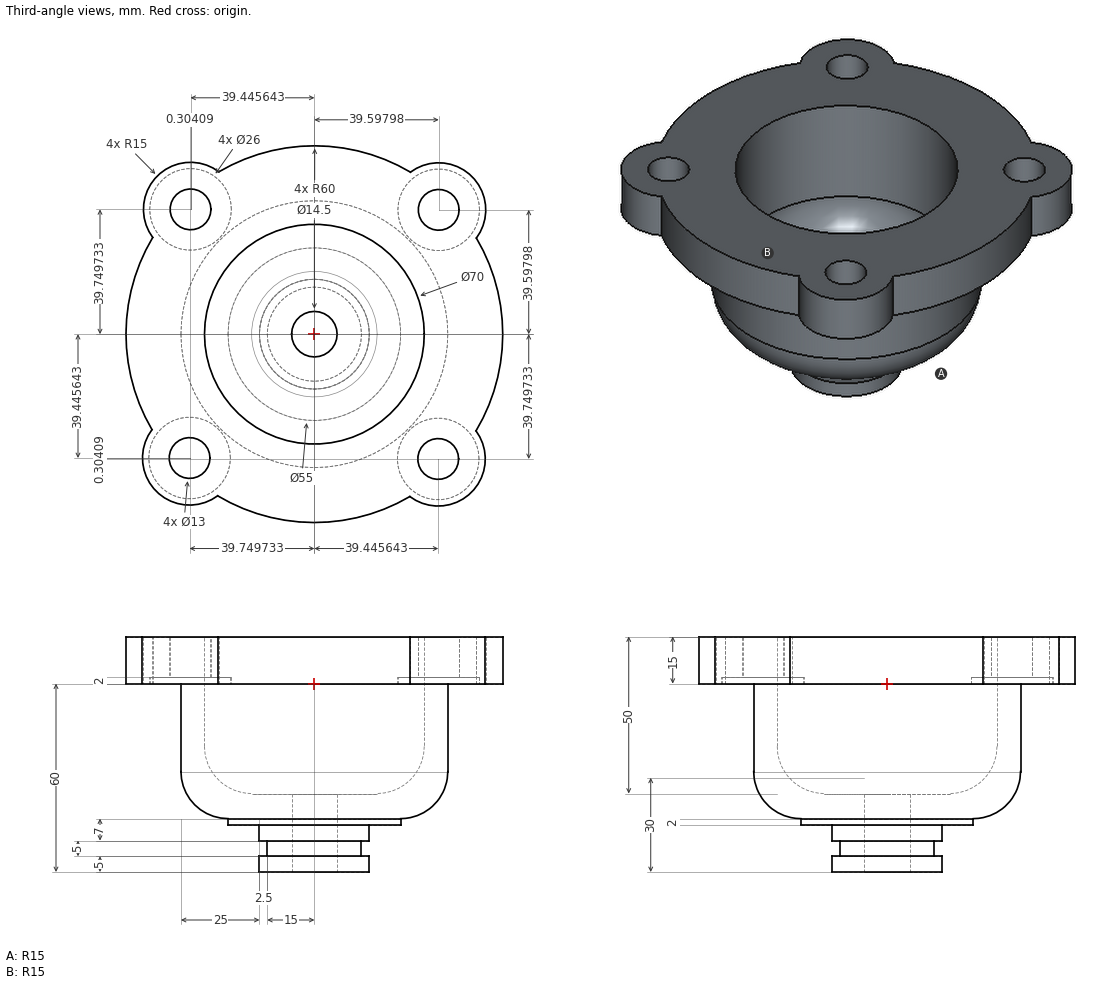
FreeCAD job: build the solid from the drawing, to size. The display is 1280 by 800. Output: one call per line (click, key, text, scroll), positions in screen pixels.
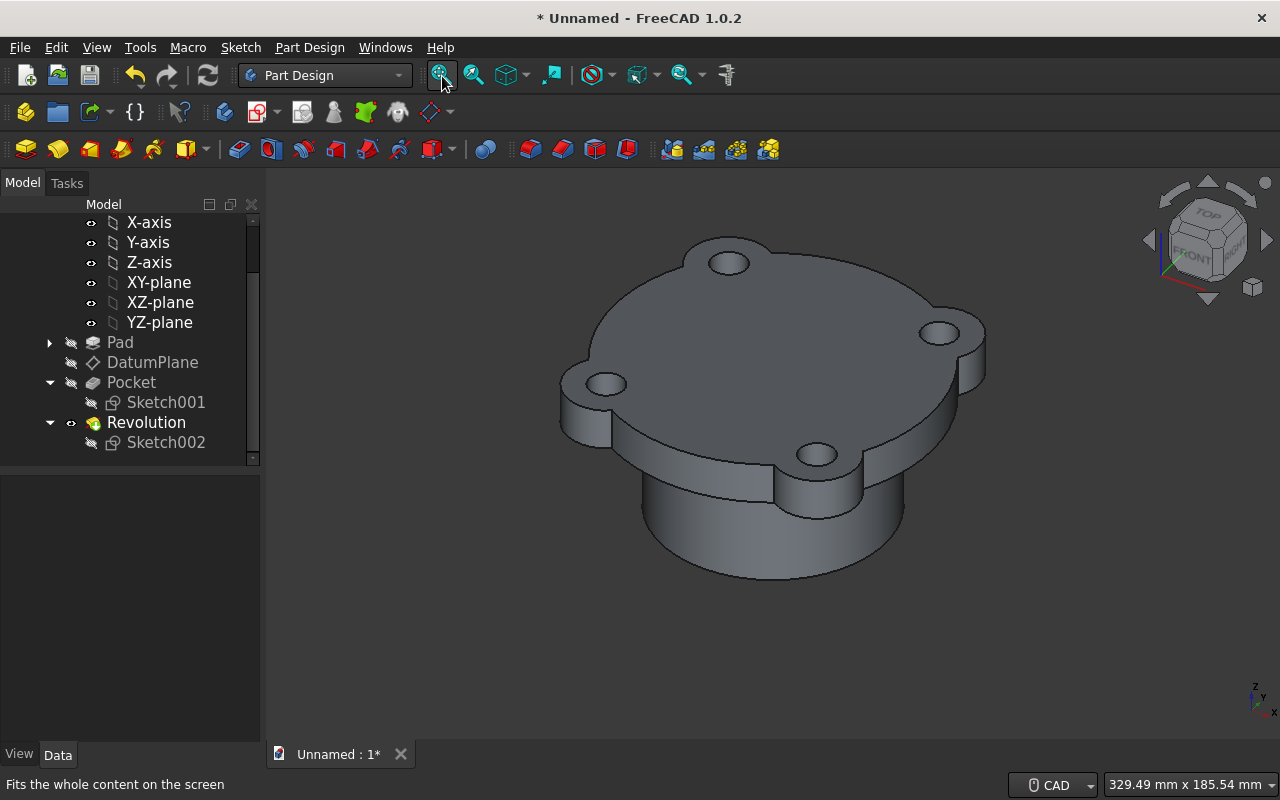
key(0)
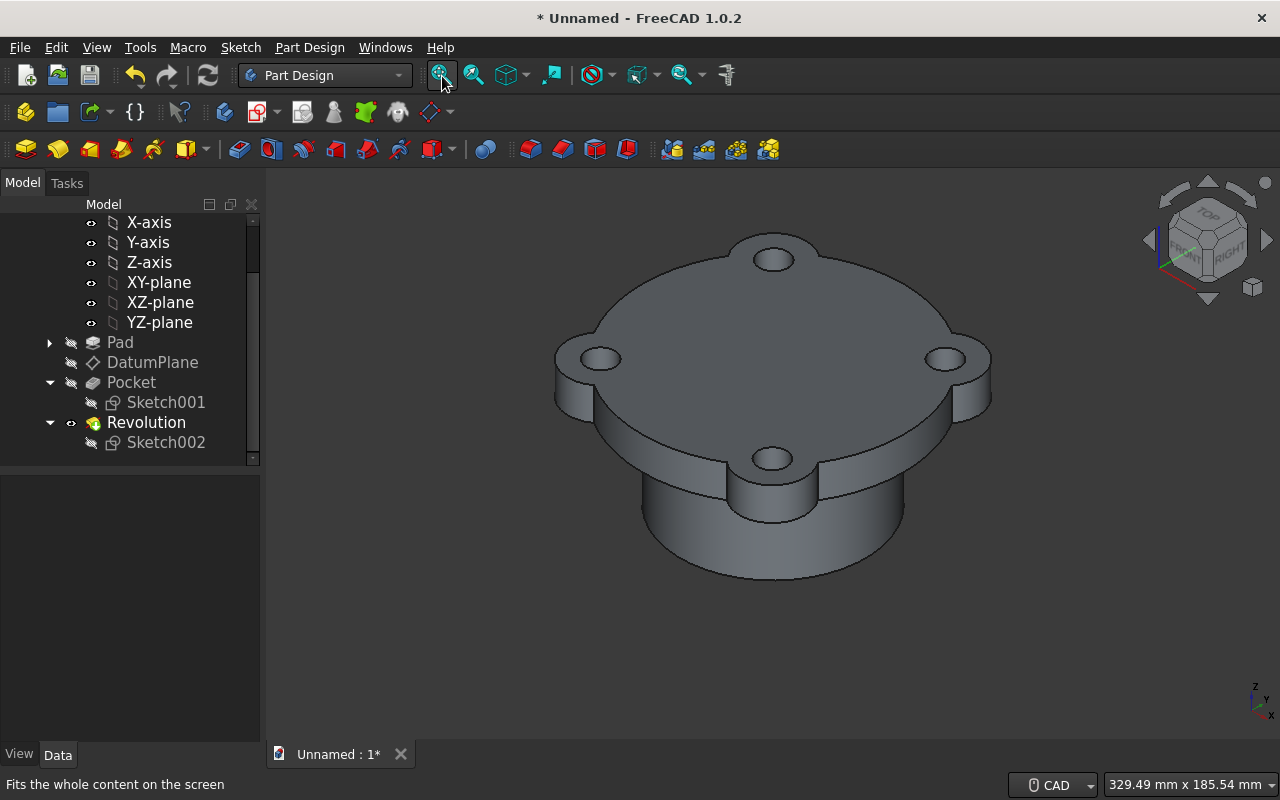
key(2)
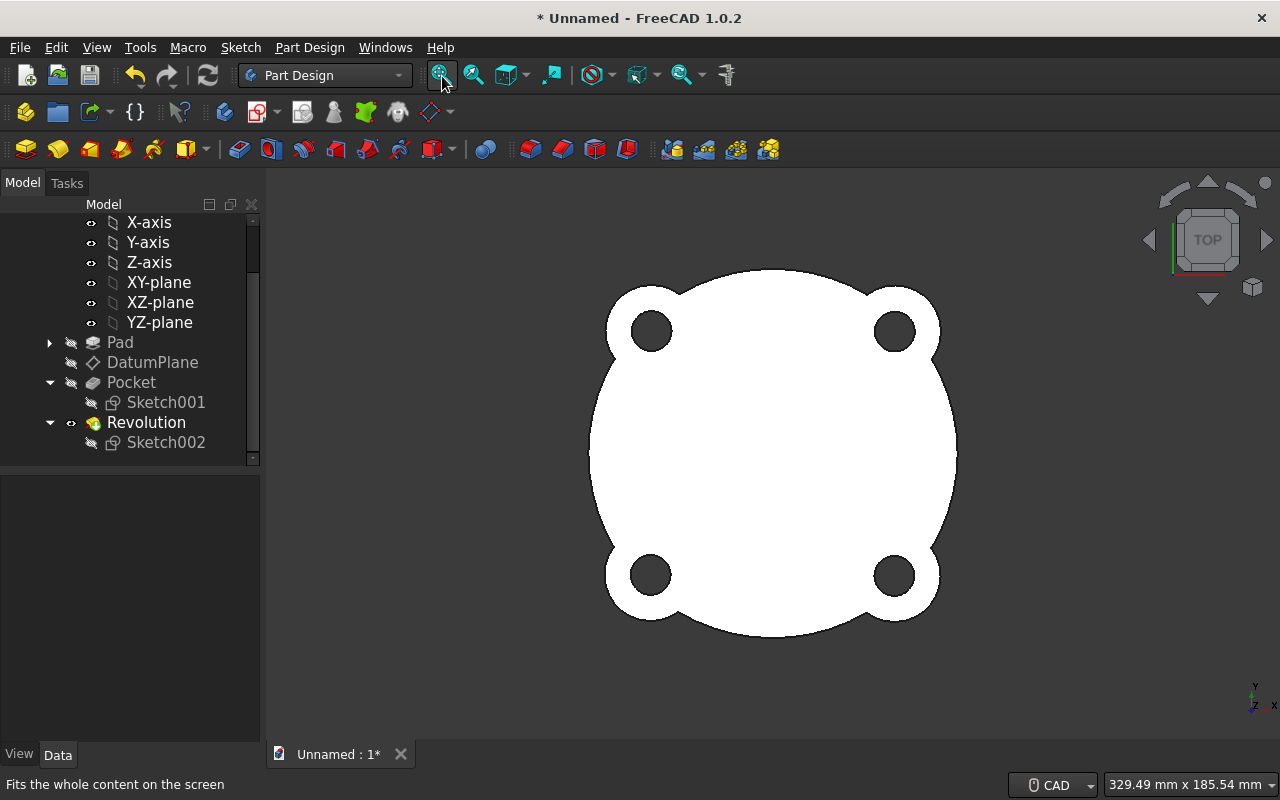
key(1)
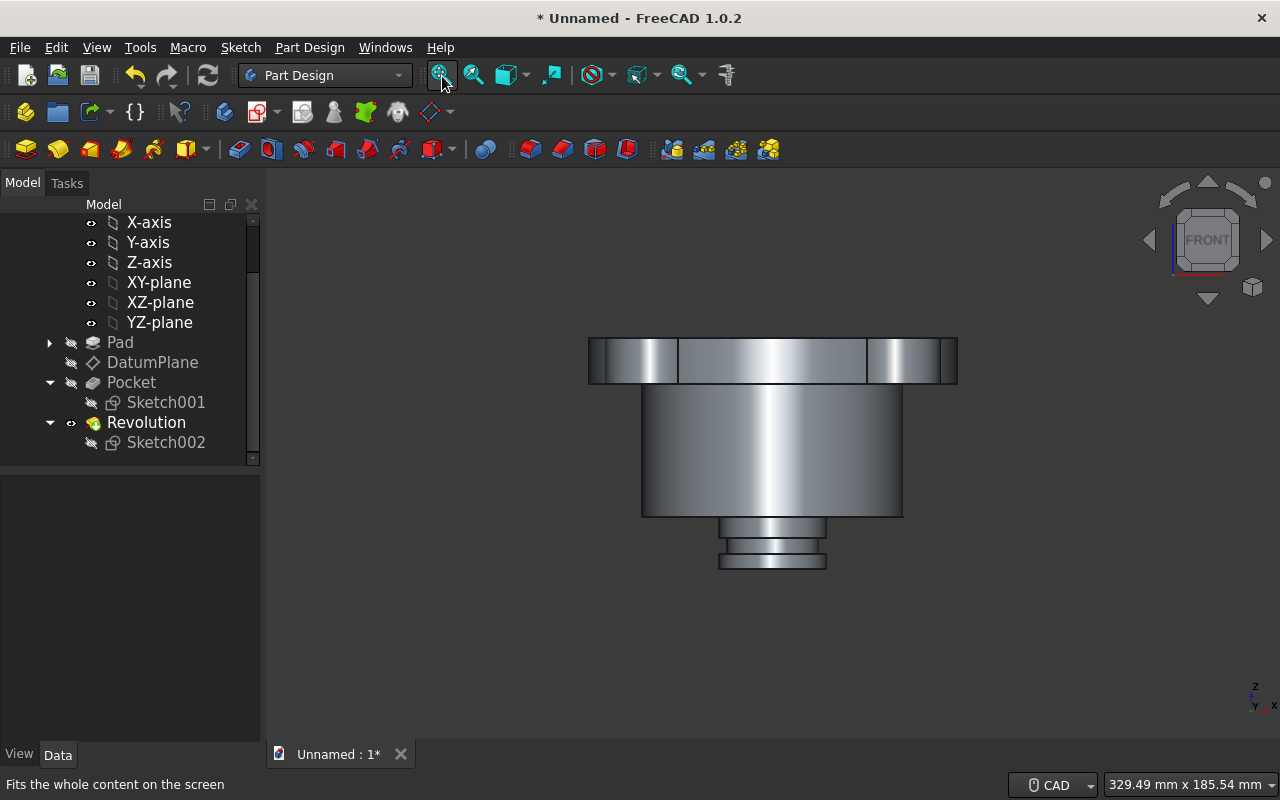
click(442, 76)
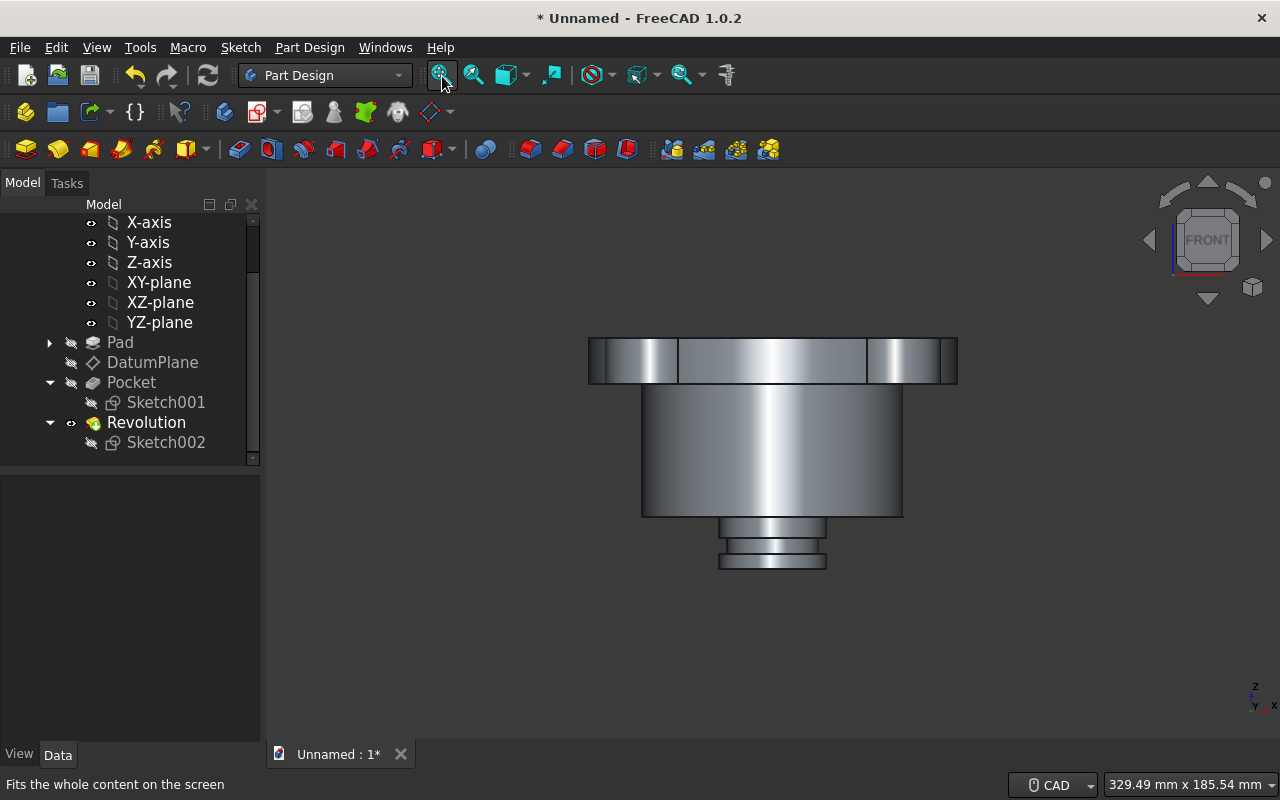
click(879, 516)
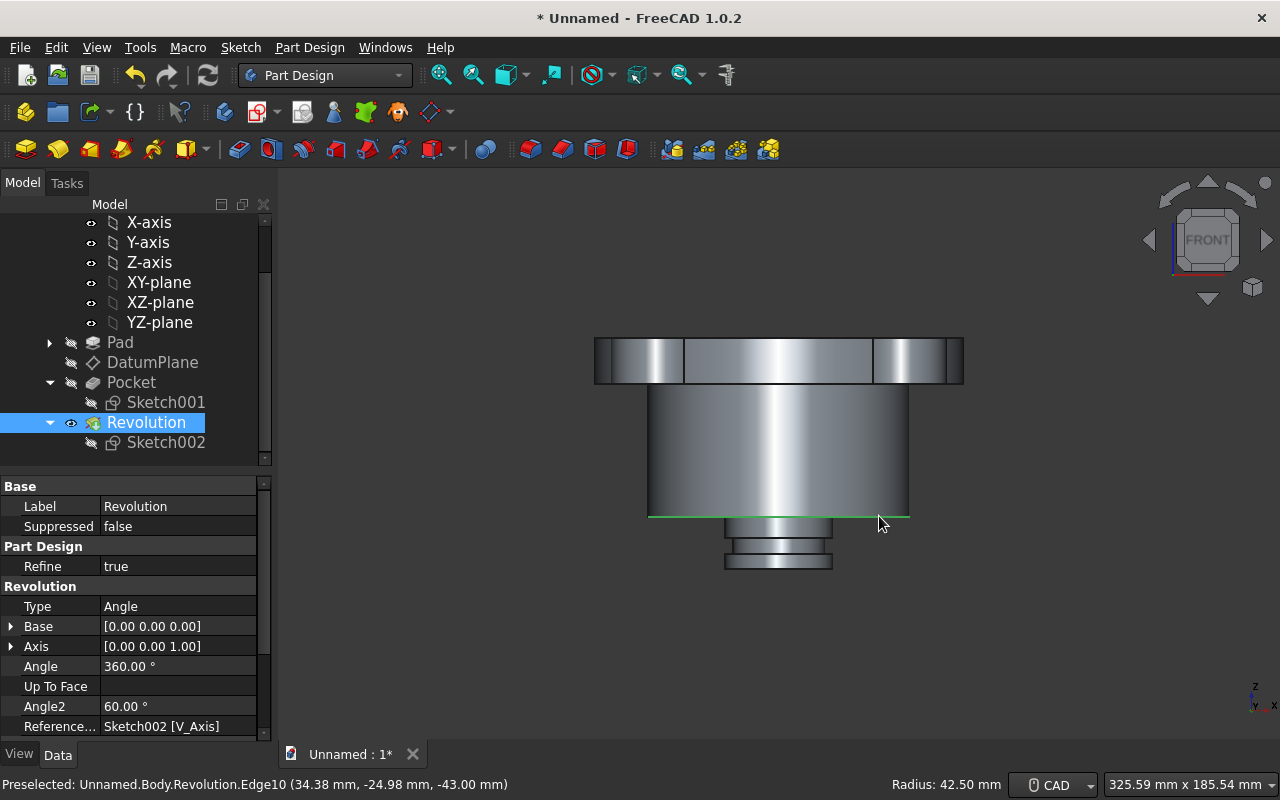
click(532, 150)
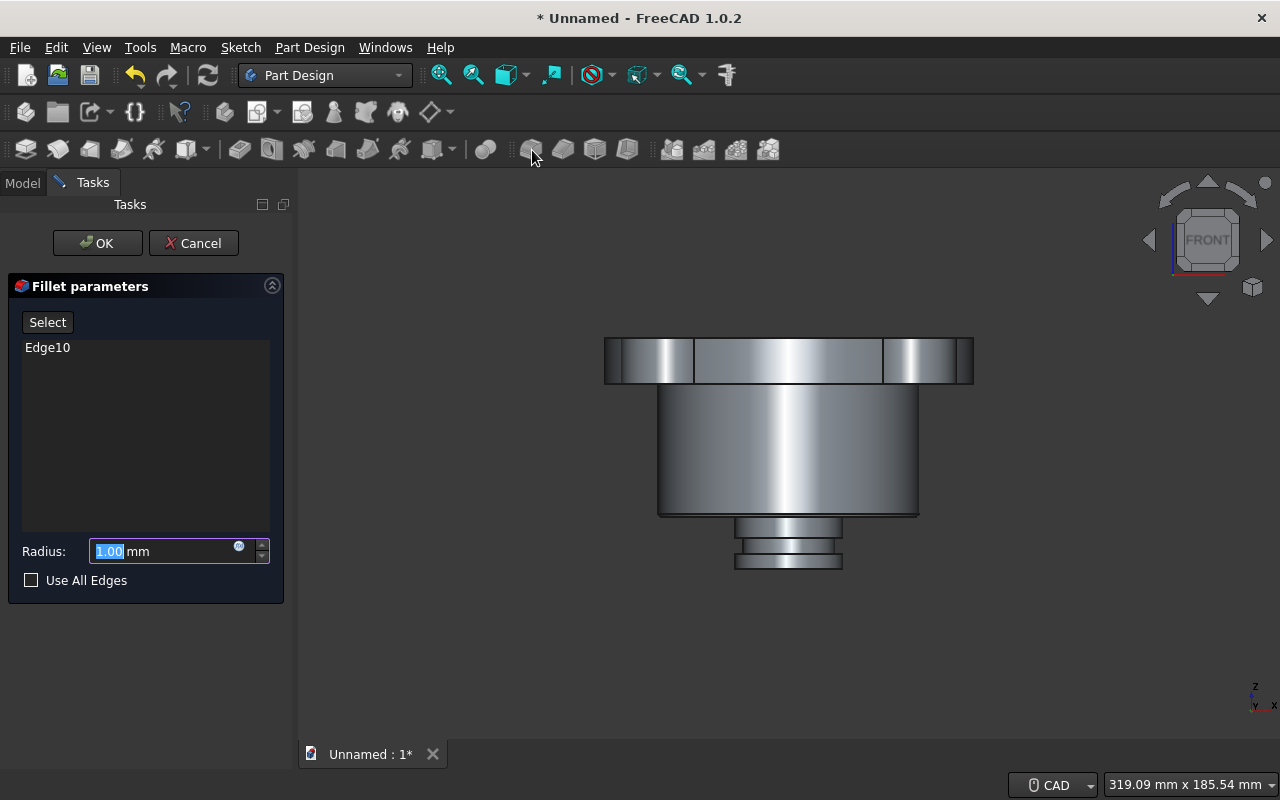
text(15)
key(Tab)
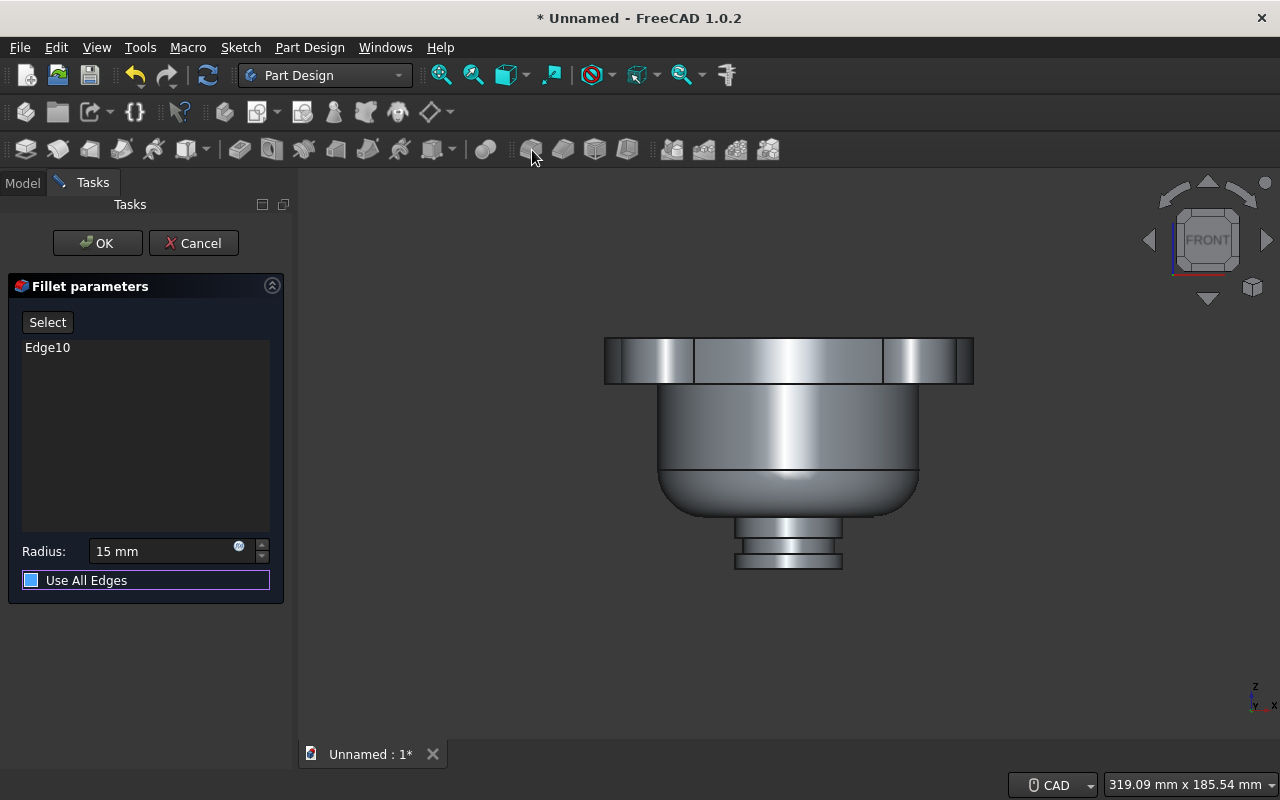
click(98, 243)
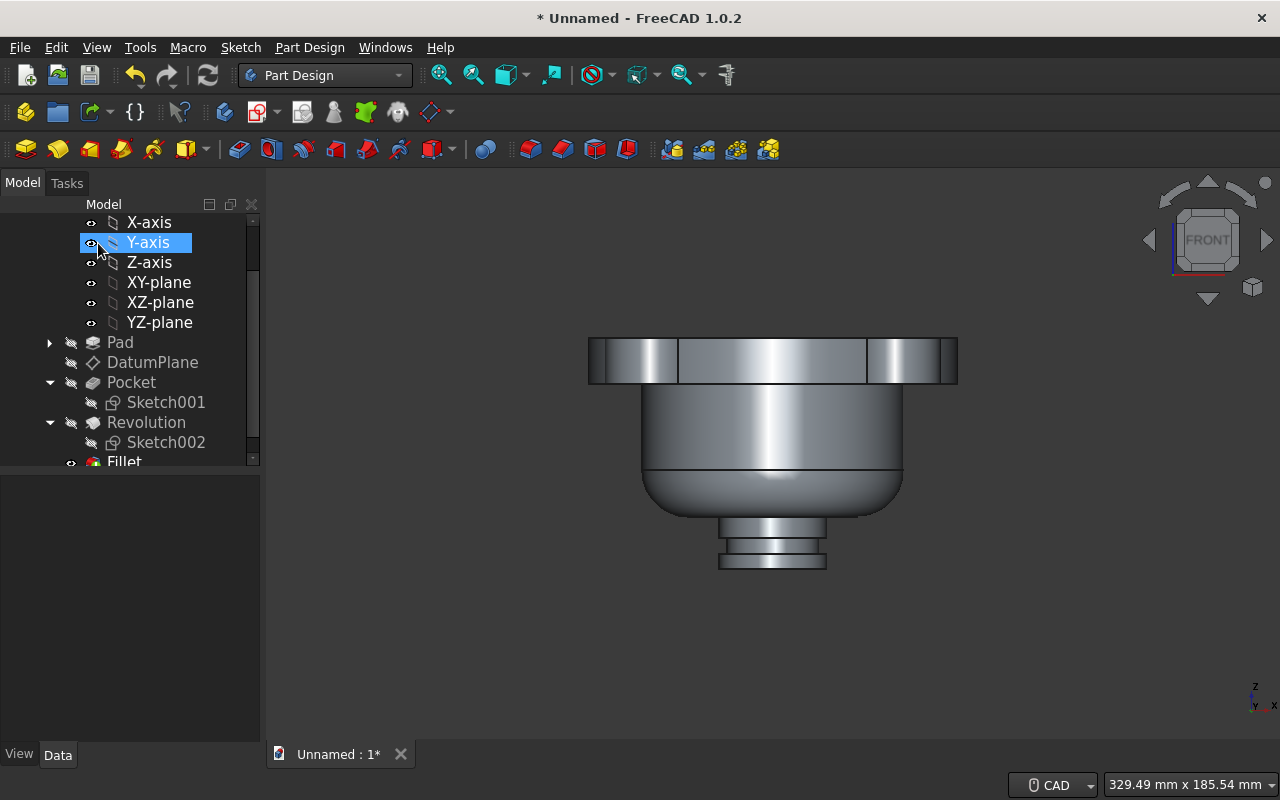
click(442, 76)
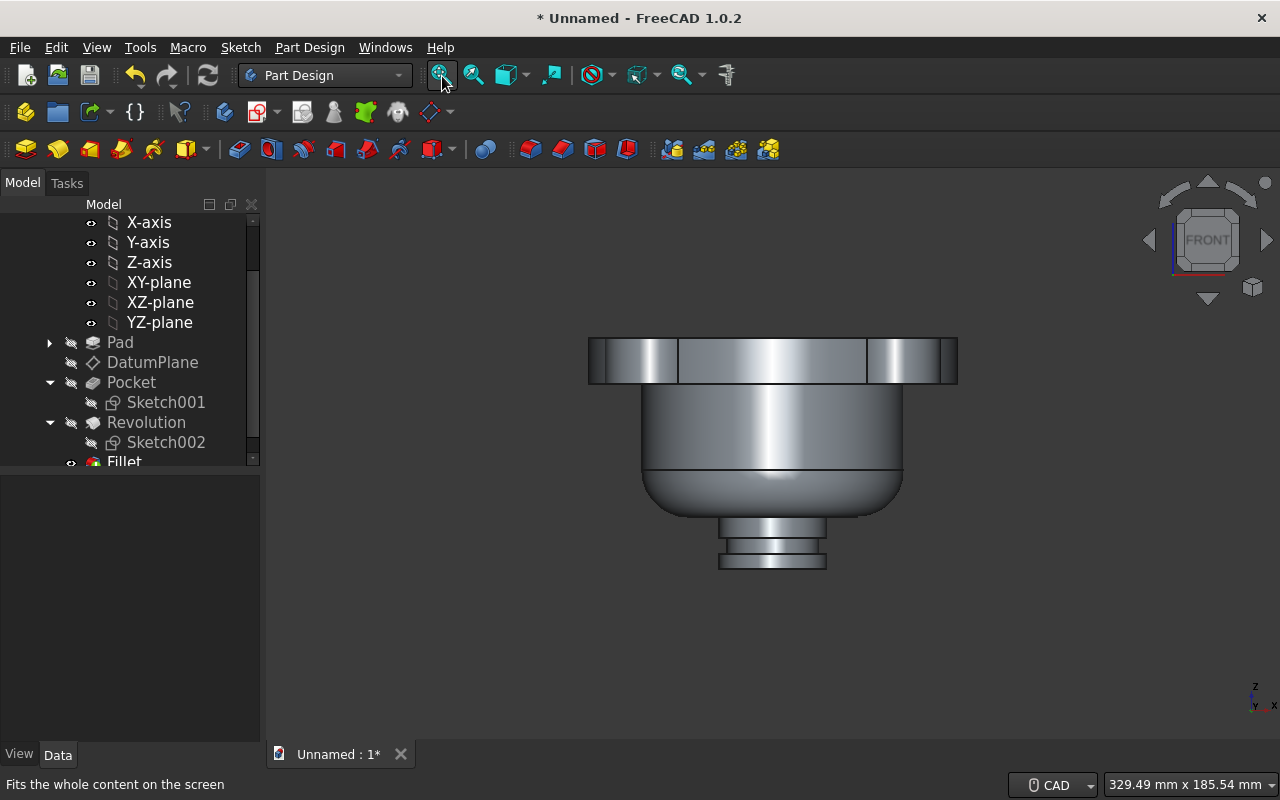
key(5)